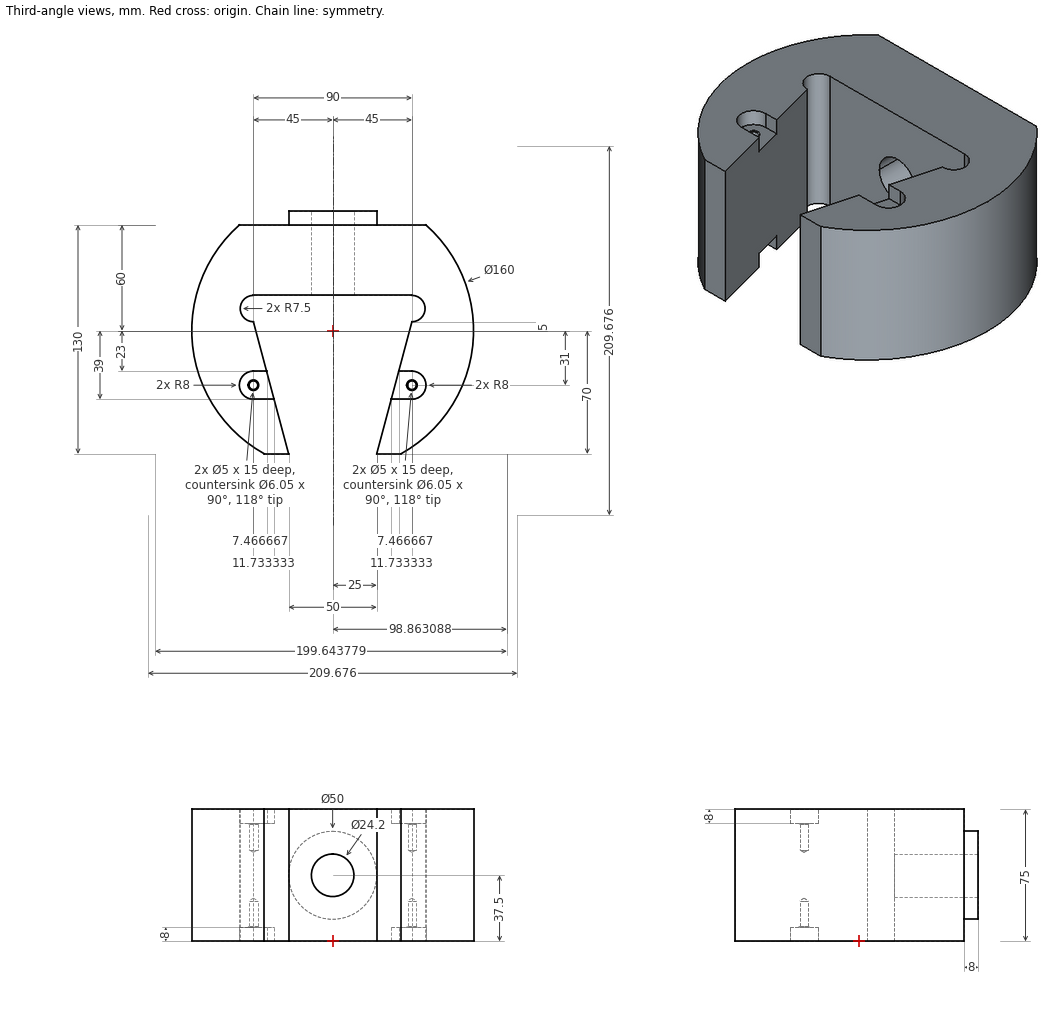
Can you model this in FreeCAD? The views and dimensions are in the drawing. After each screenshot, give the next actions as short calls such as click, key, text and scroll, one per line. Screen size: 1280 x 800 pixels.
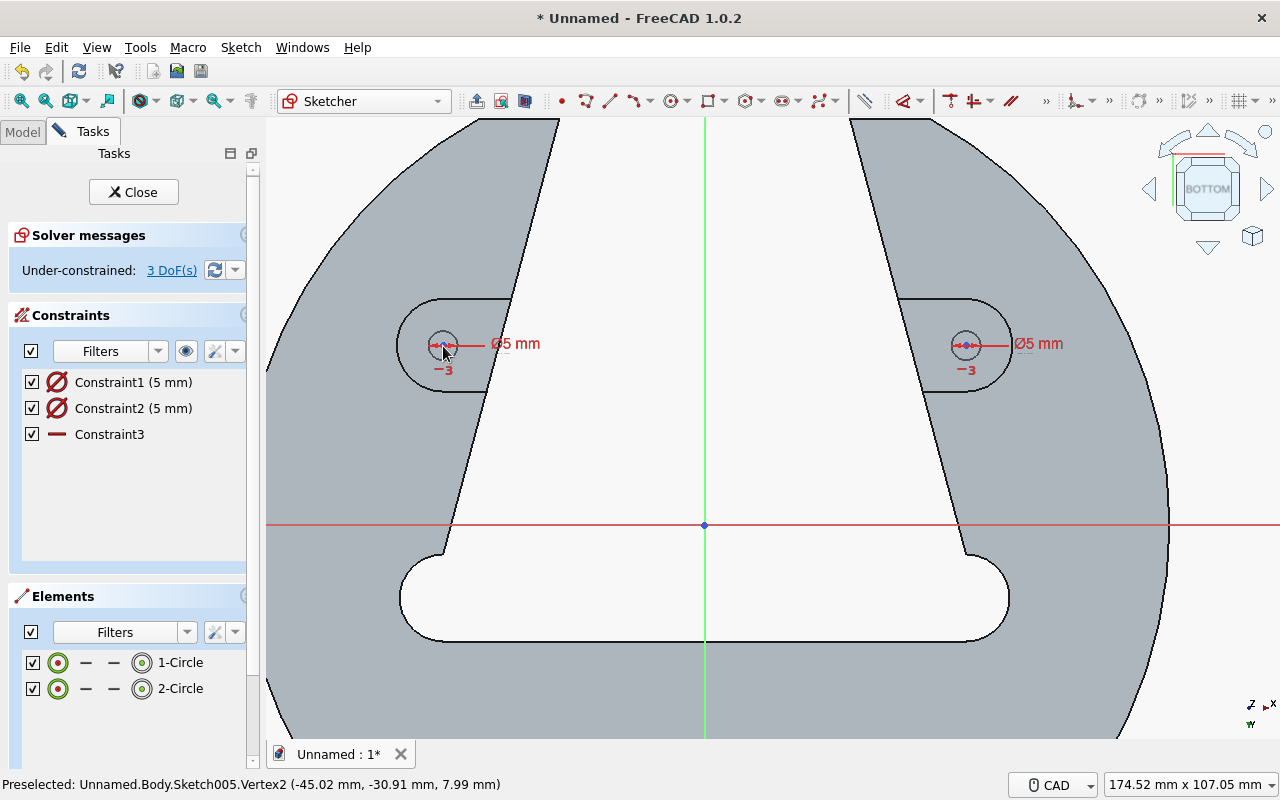
key(d)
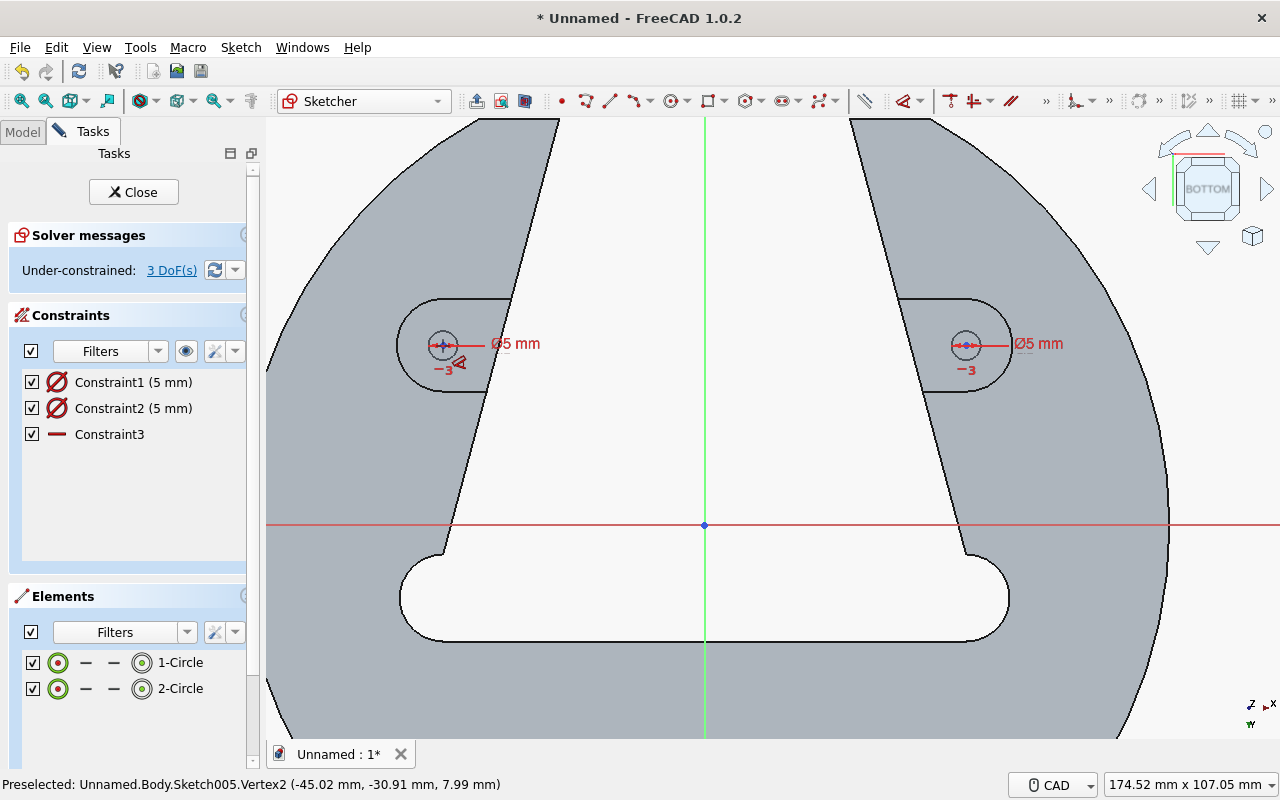
click(966, 346)
click(835, 559)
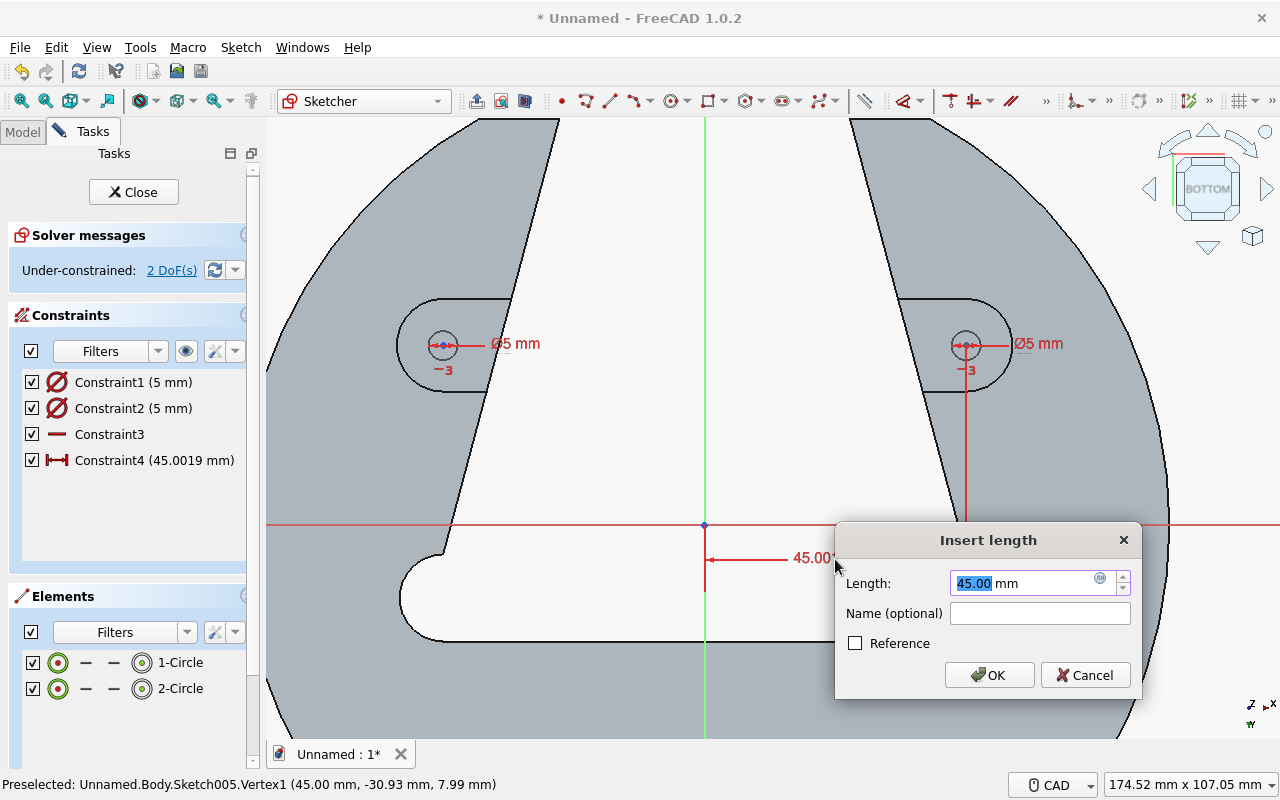
text(45)
key(Return)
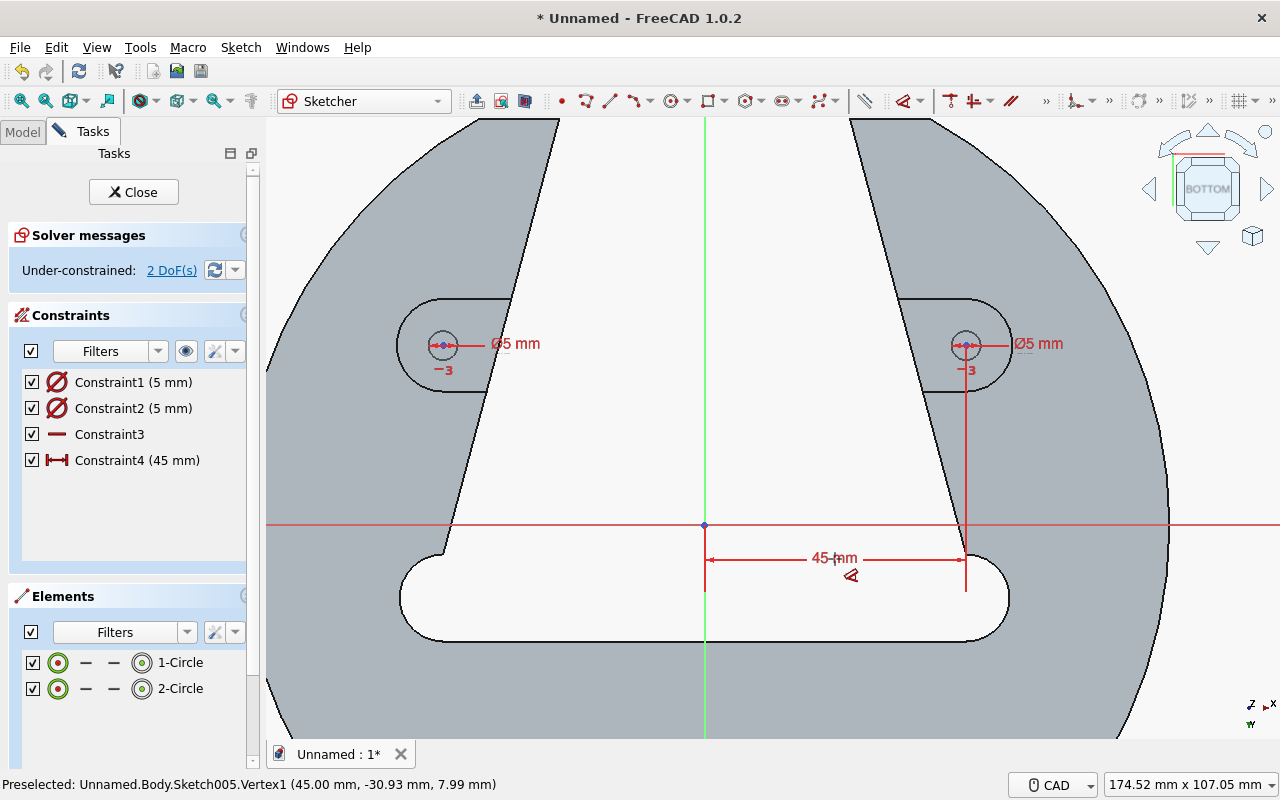
click(966, 346)
click(1000, 435)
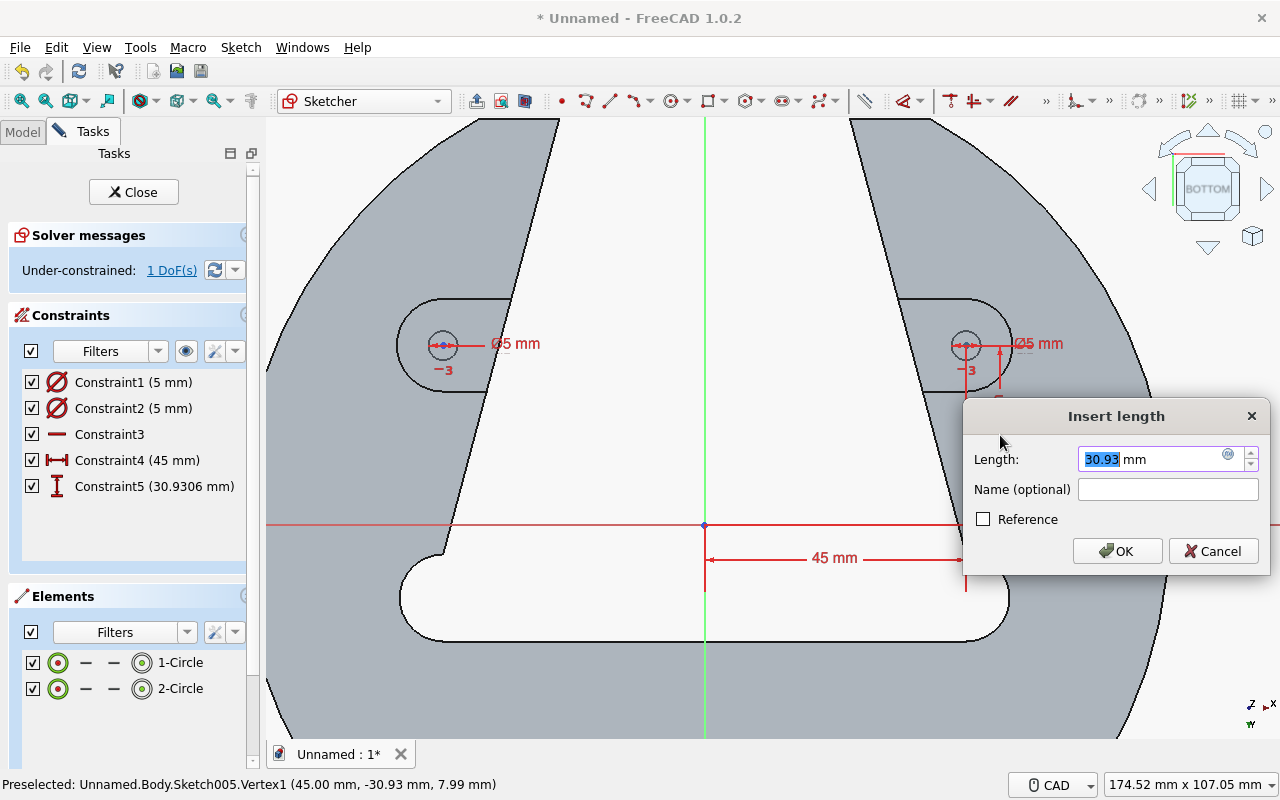
text(31)
key(Return)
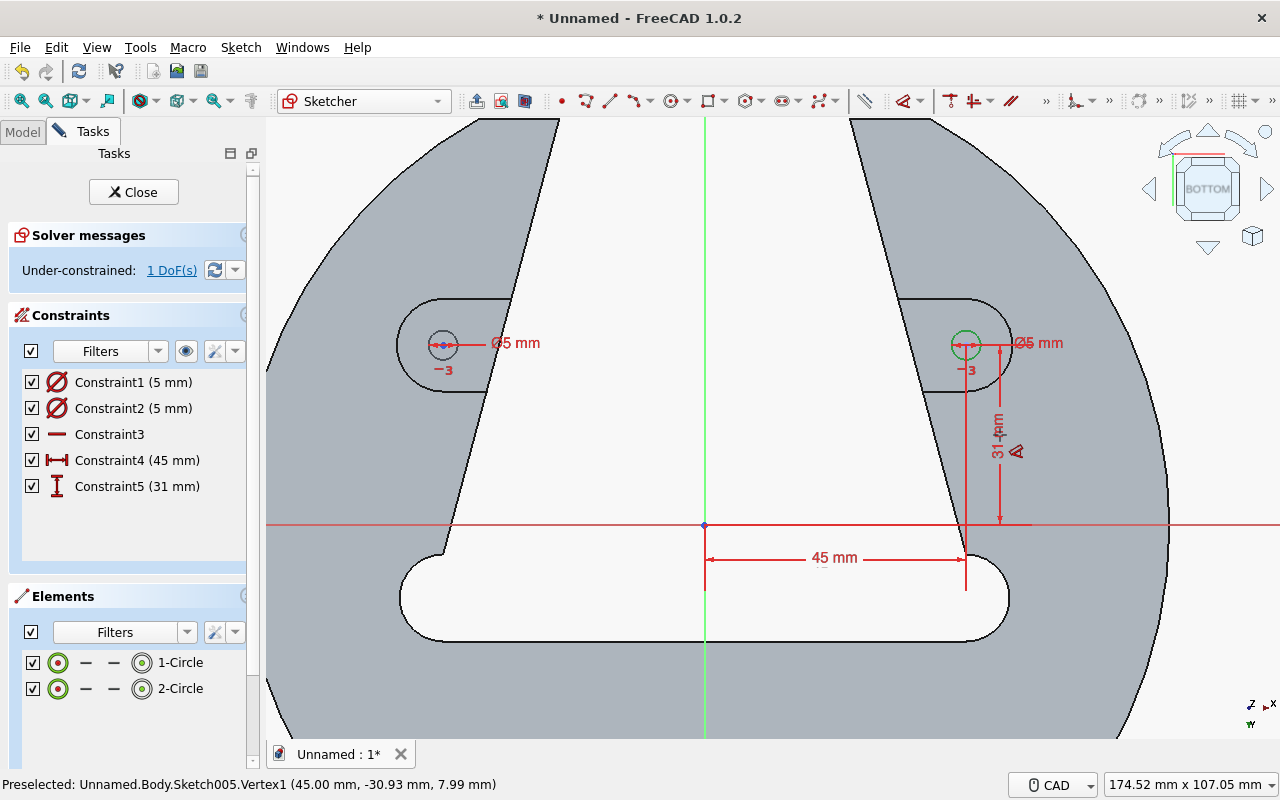
click(443, 345)
click(574, 559)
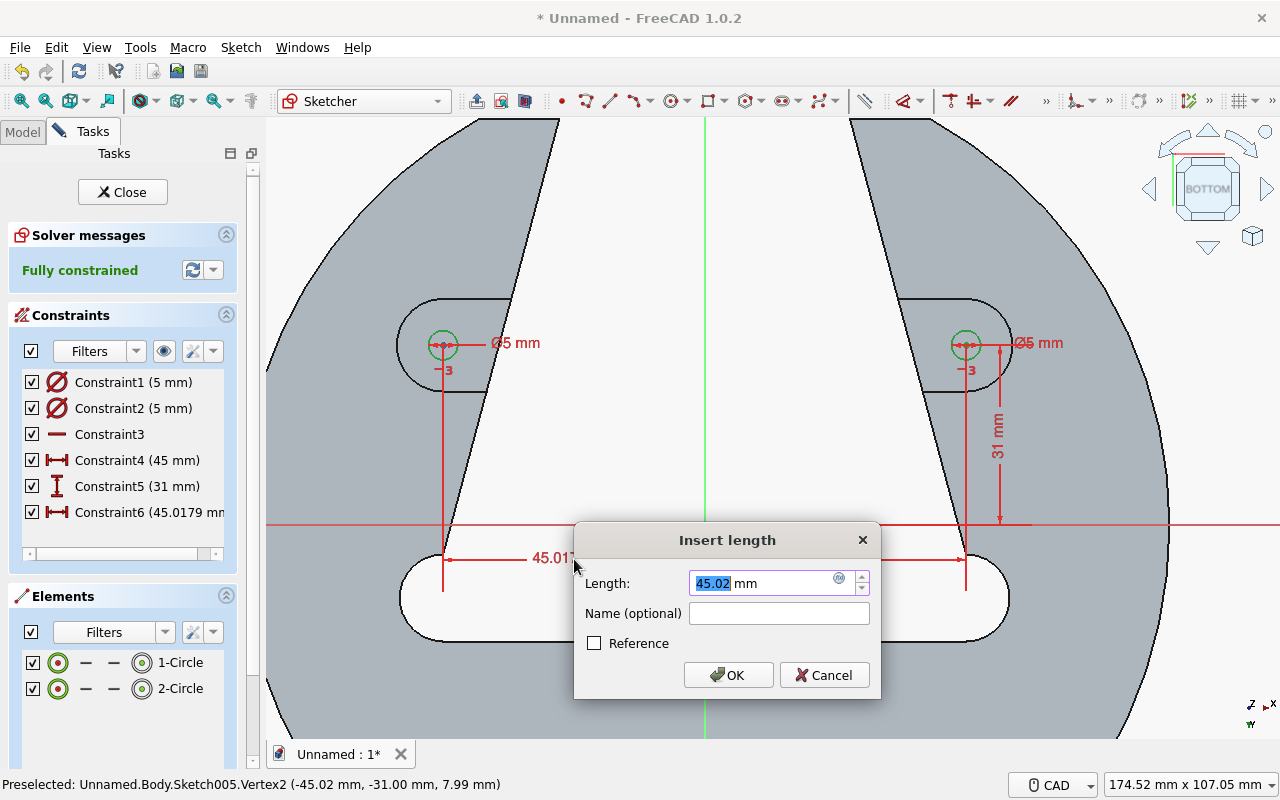
text(45)
key(Return)
key(Escape)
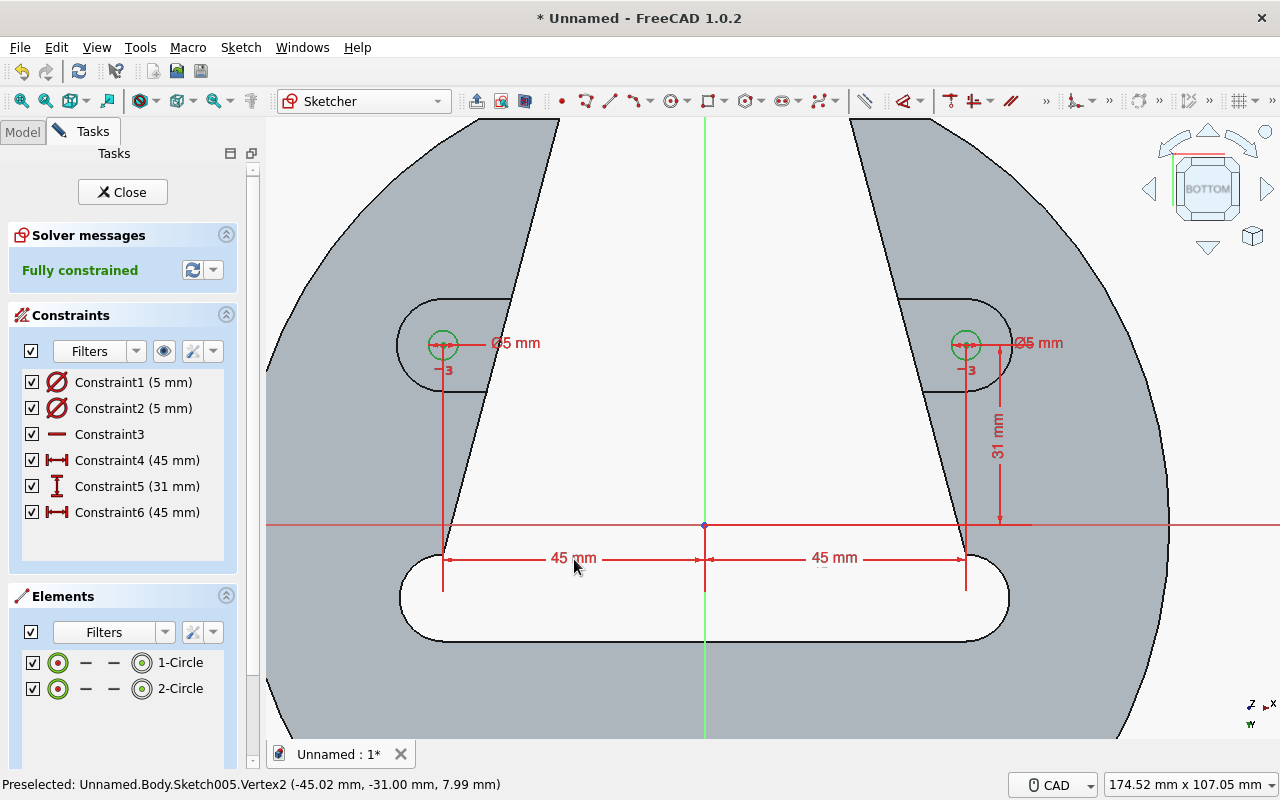
click(123, 192)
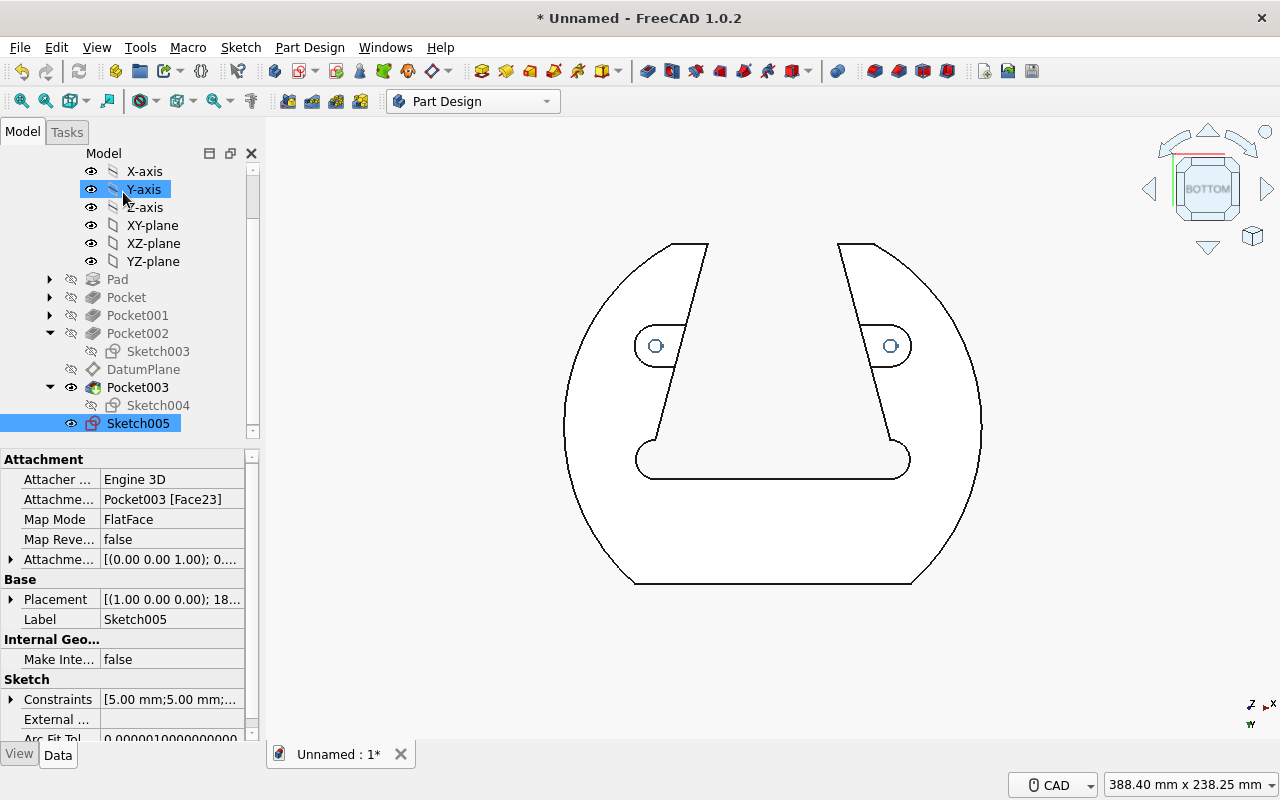
click(672, 72)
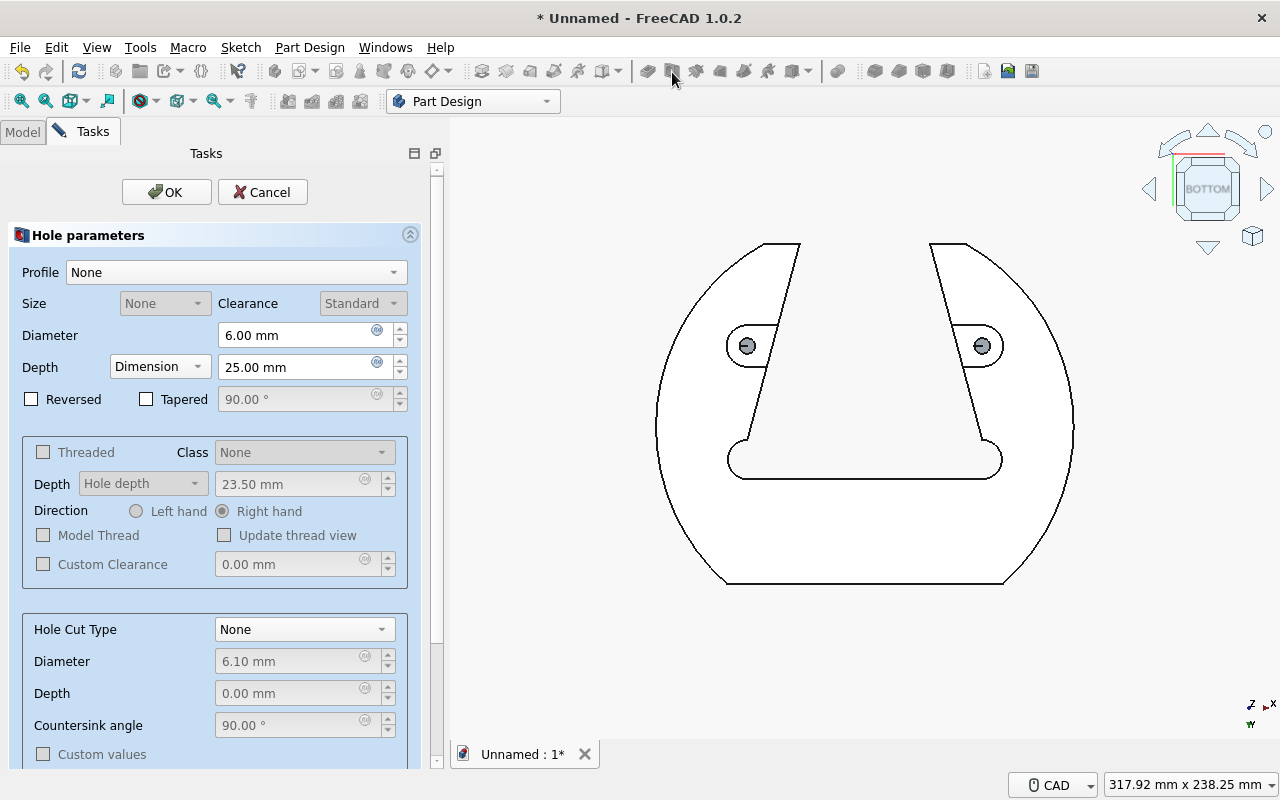
triple_click(305, 335)